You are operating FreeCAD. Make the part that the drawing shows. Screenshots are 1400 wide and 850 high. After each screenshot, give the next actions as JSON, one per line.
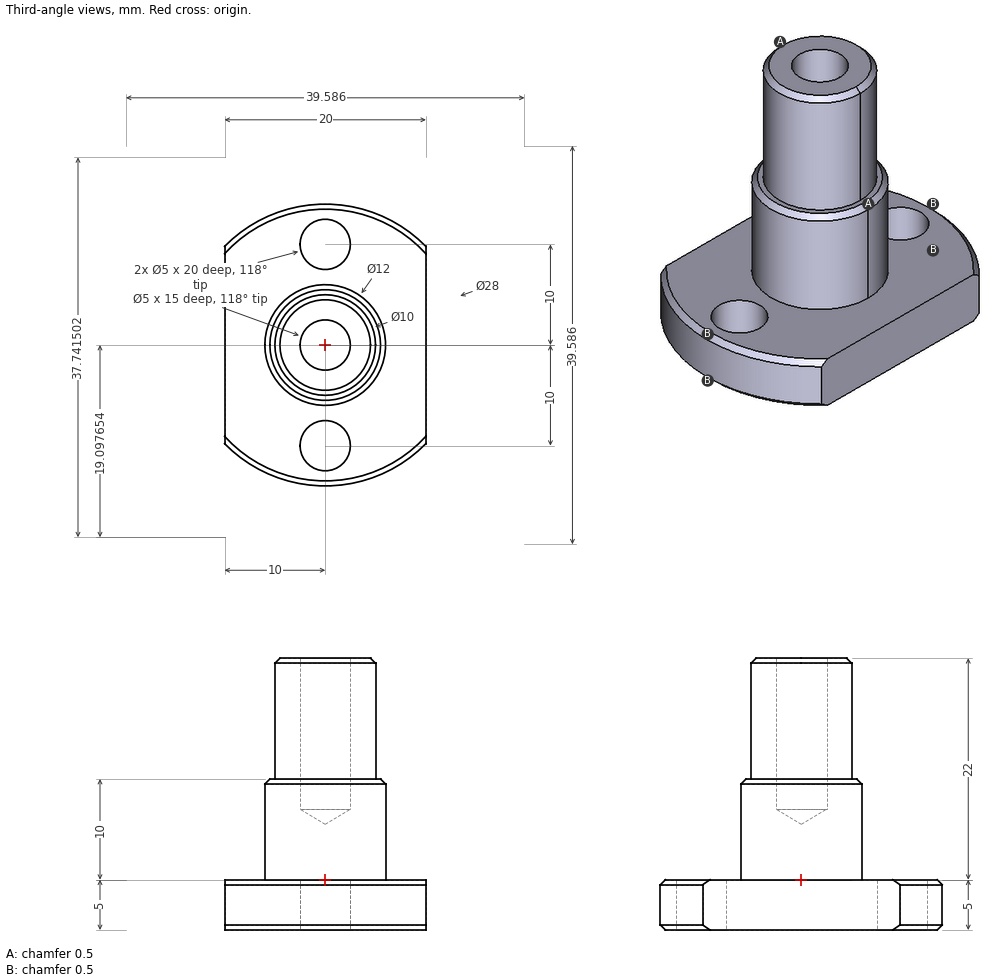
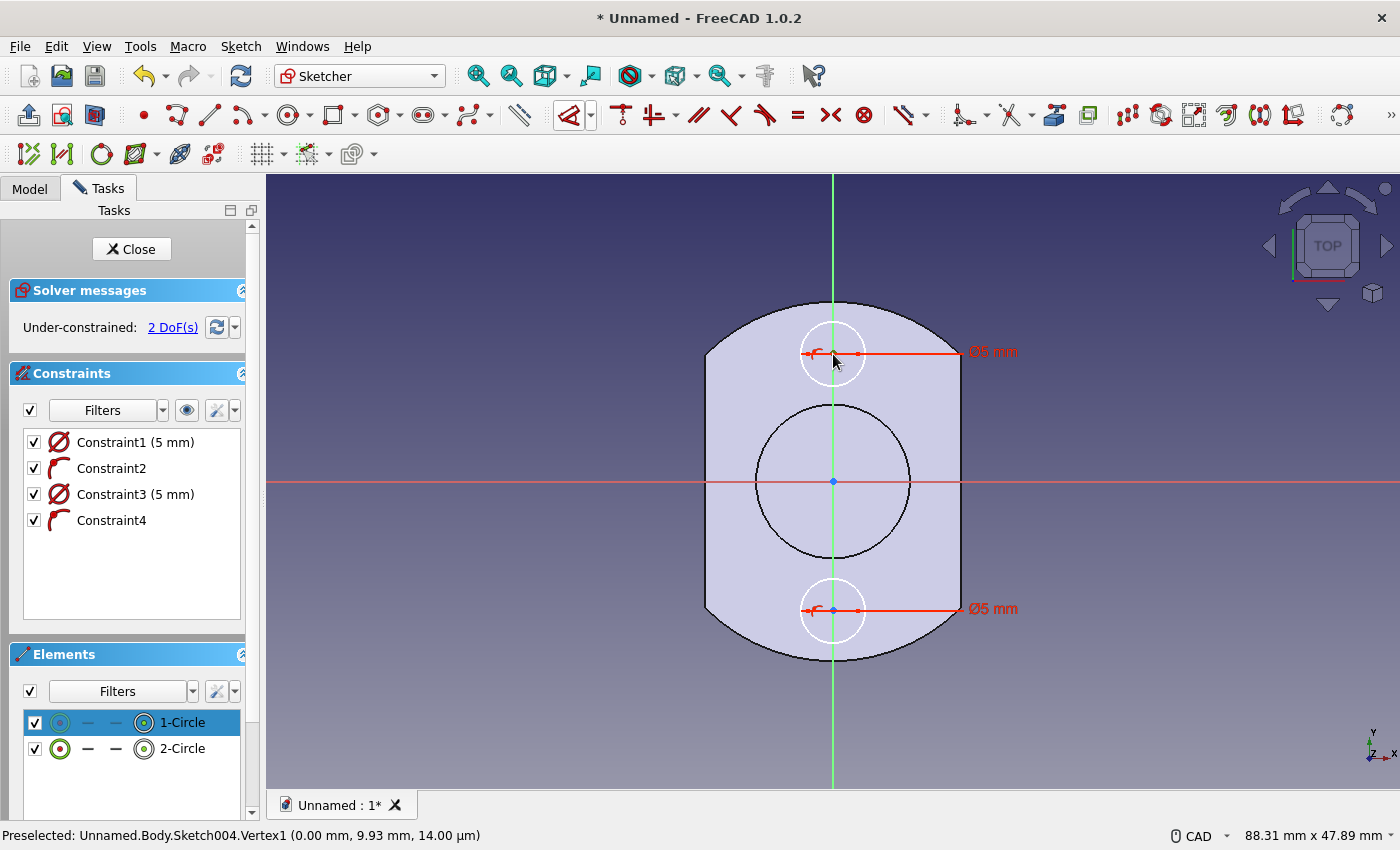
{"action": "key", "text": "i"}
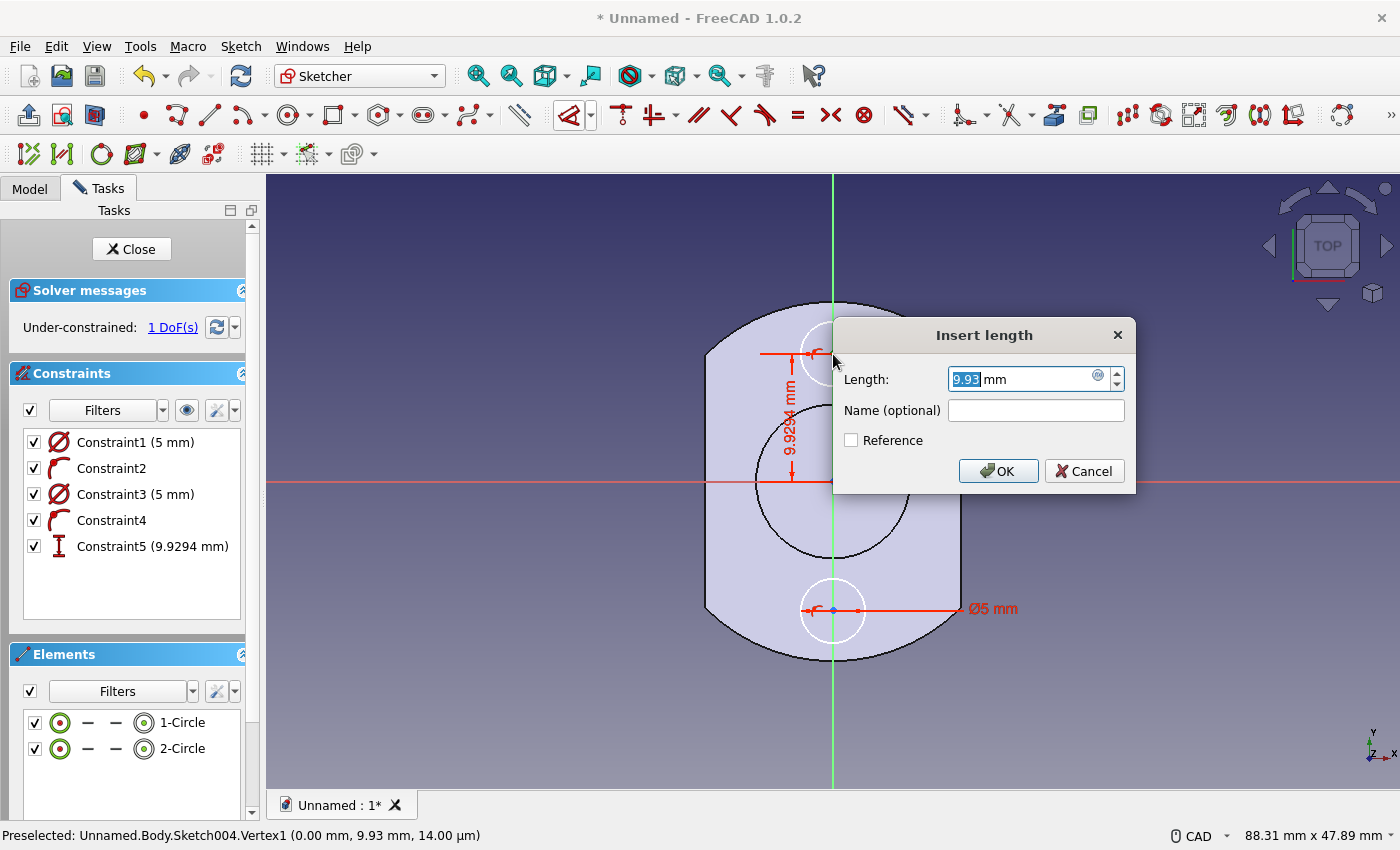
{"action": "type", "text": "10"}
{"action": "key", "text": "Return"}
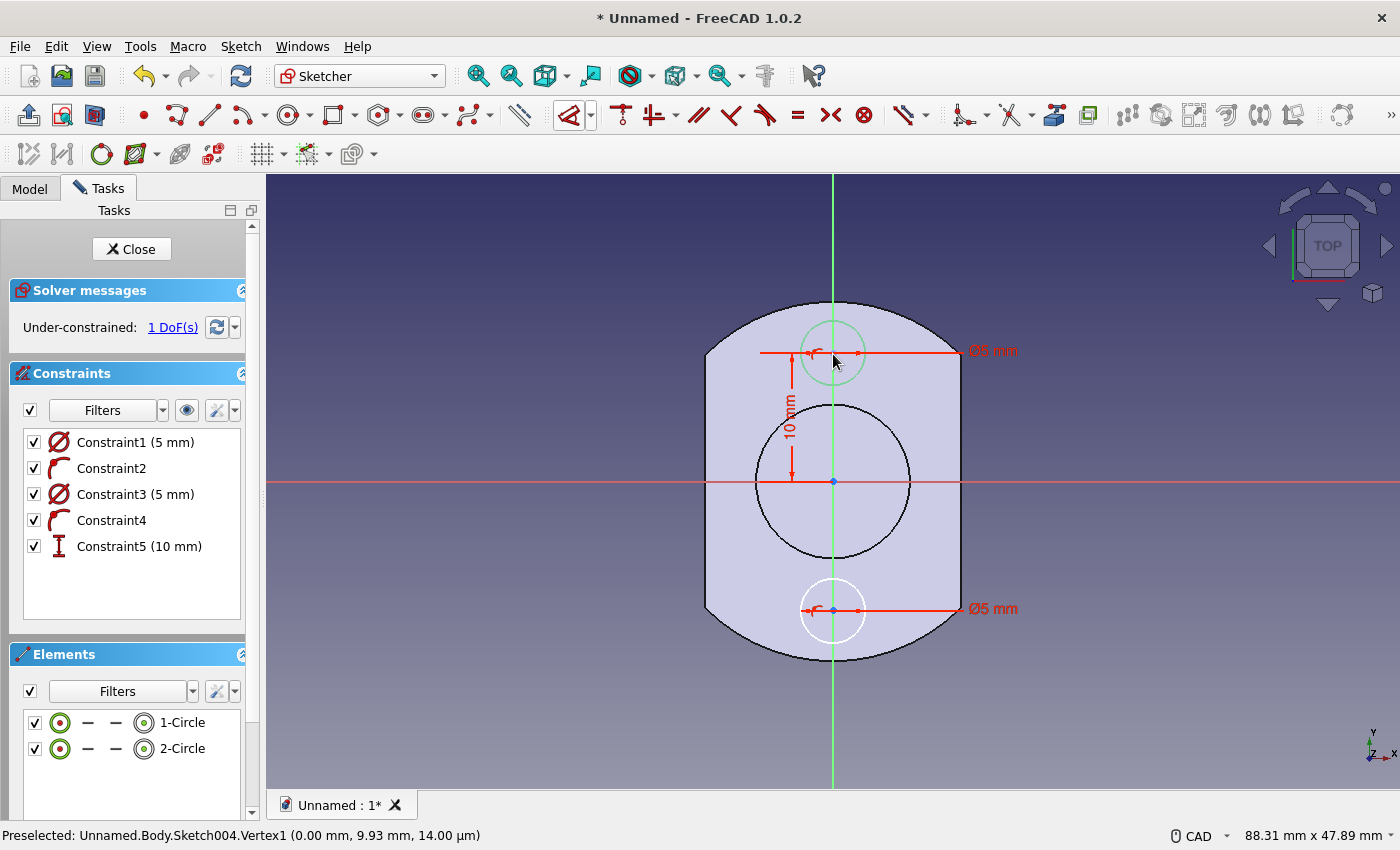
{"action": "left_click", "coordinate": [833, 611]}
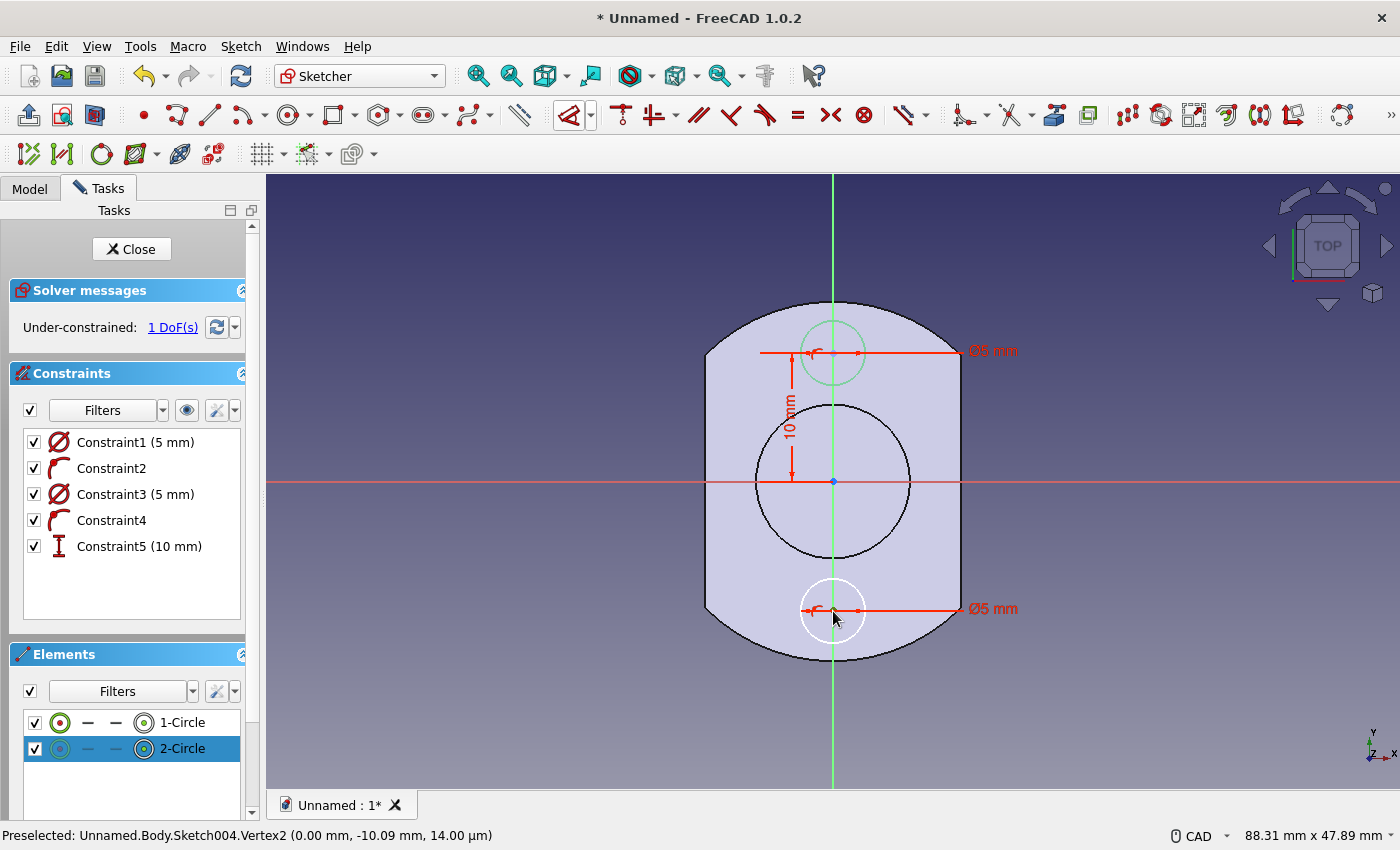
{"action": "key", "text": "i"}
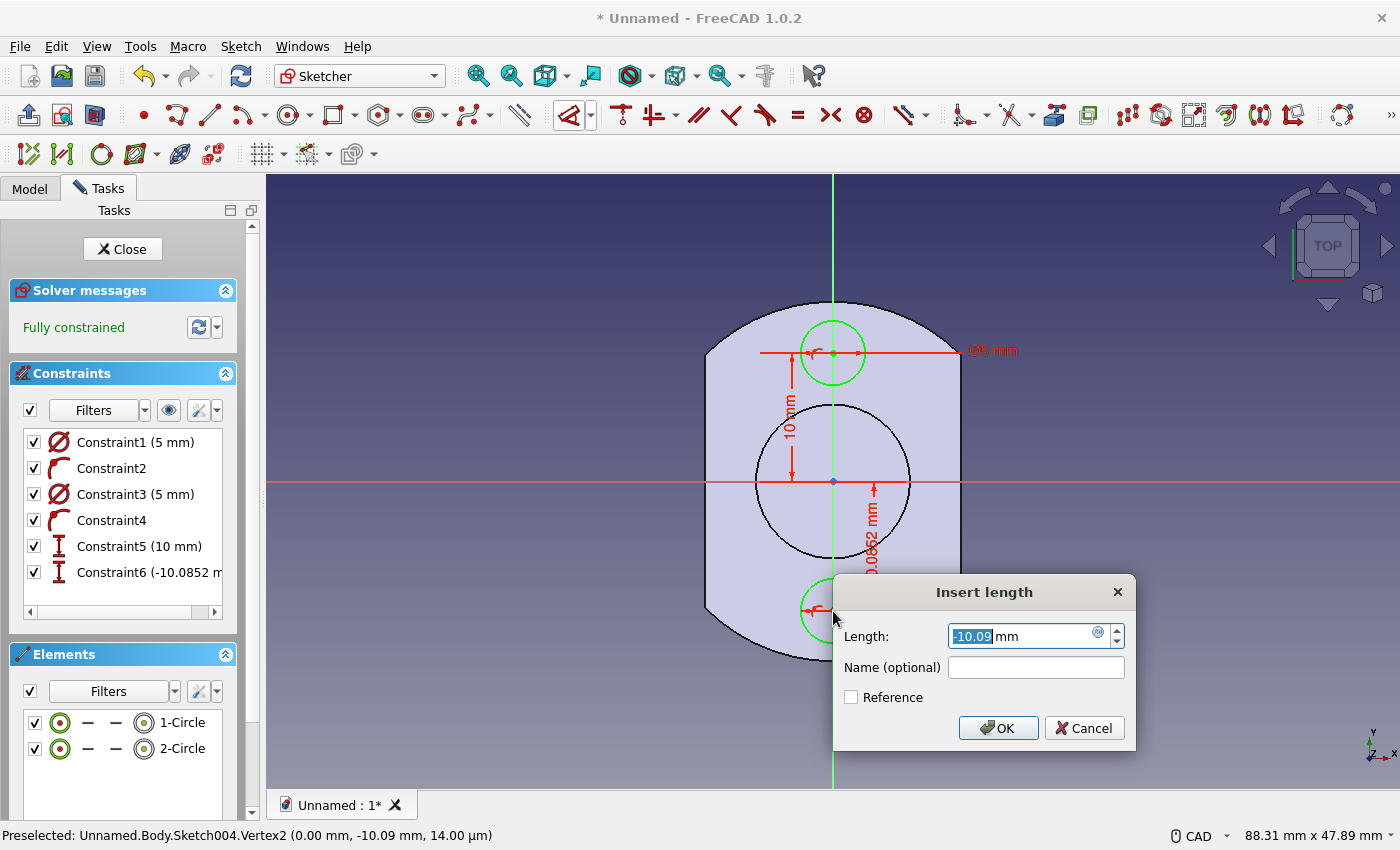
{"action": "type", "text": "-10"}
{"action": "key", "text": "Return"}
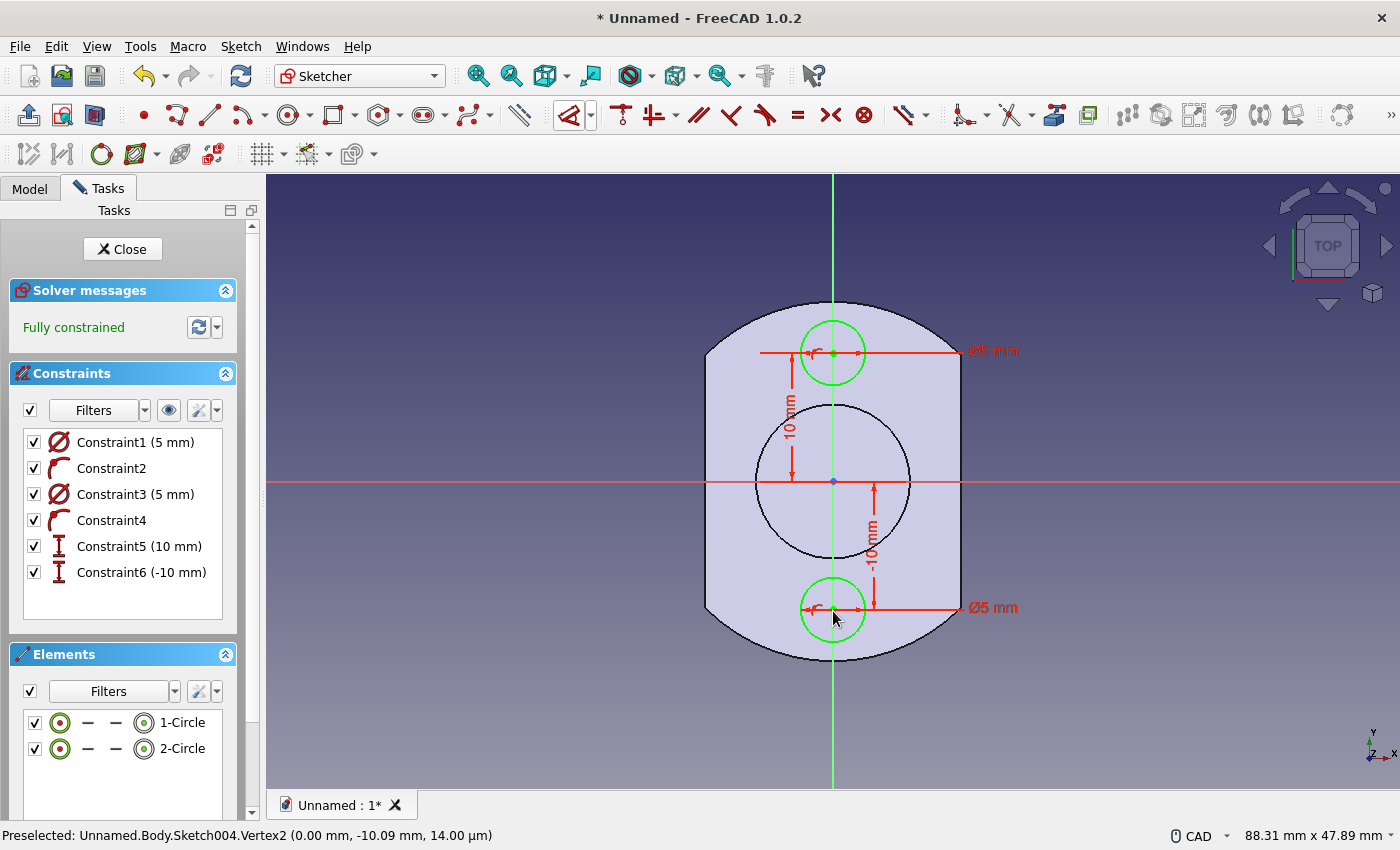
{"action": "left_click", "coordinate": [123, 249]}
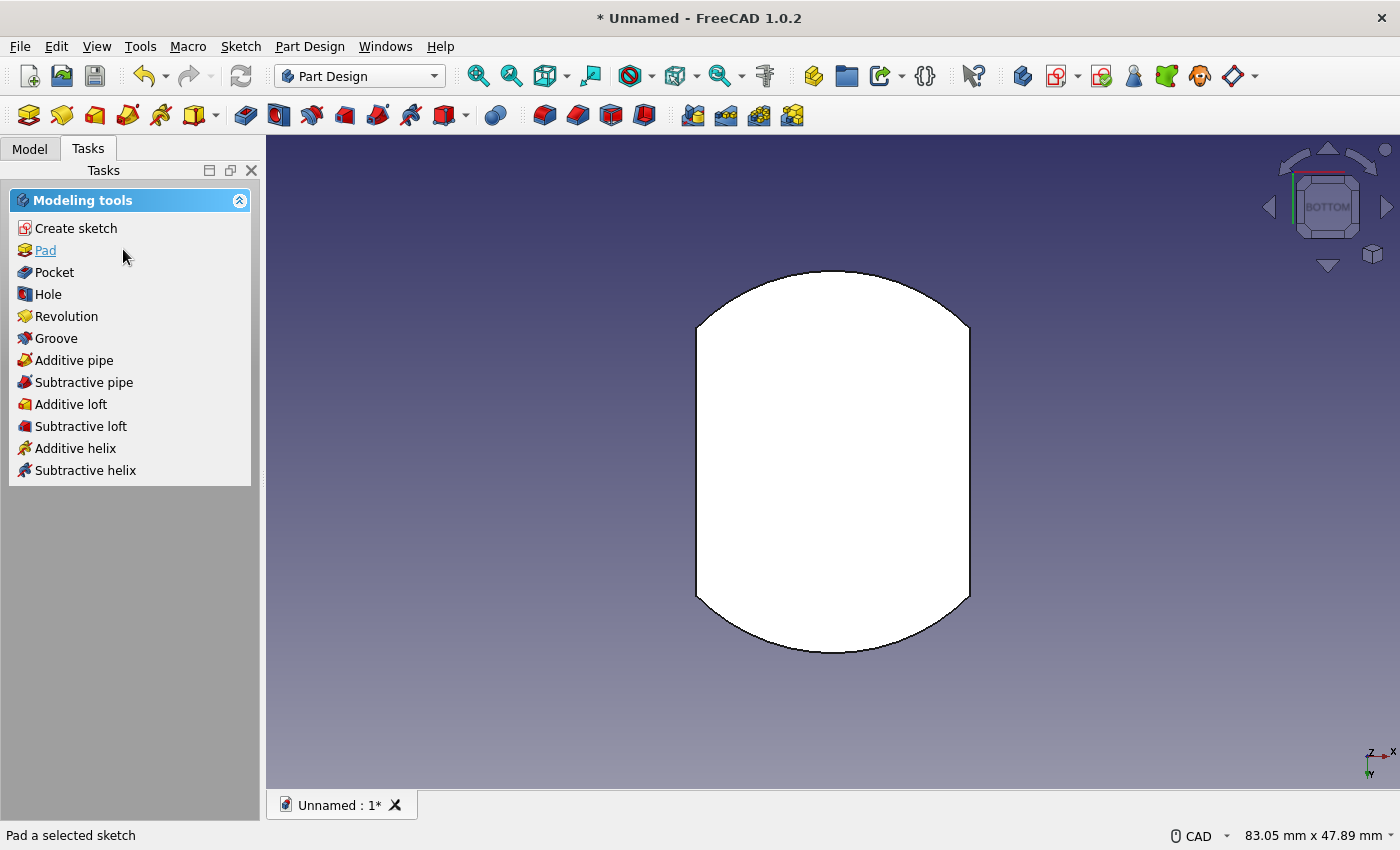
{"action": "left_click", "coordinate": [279, 116]}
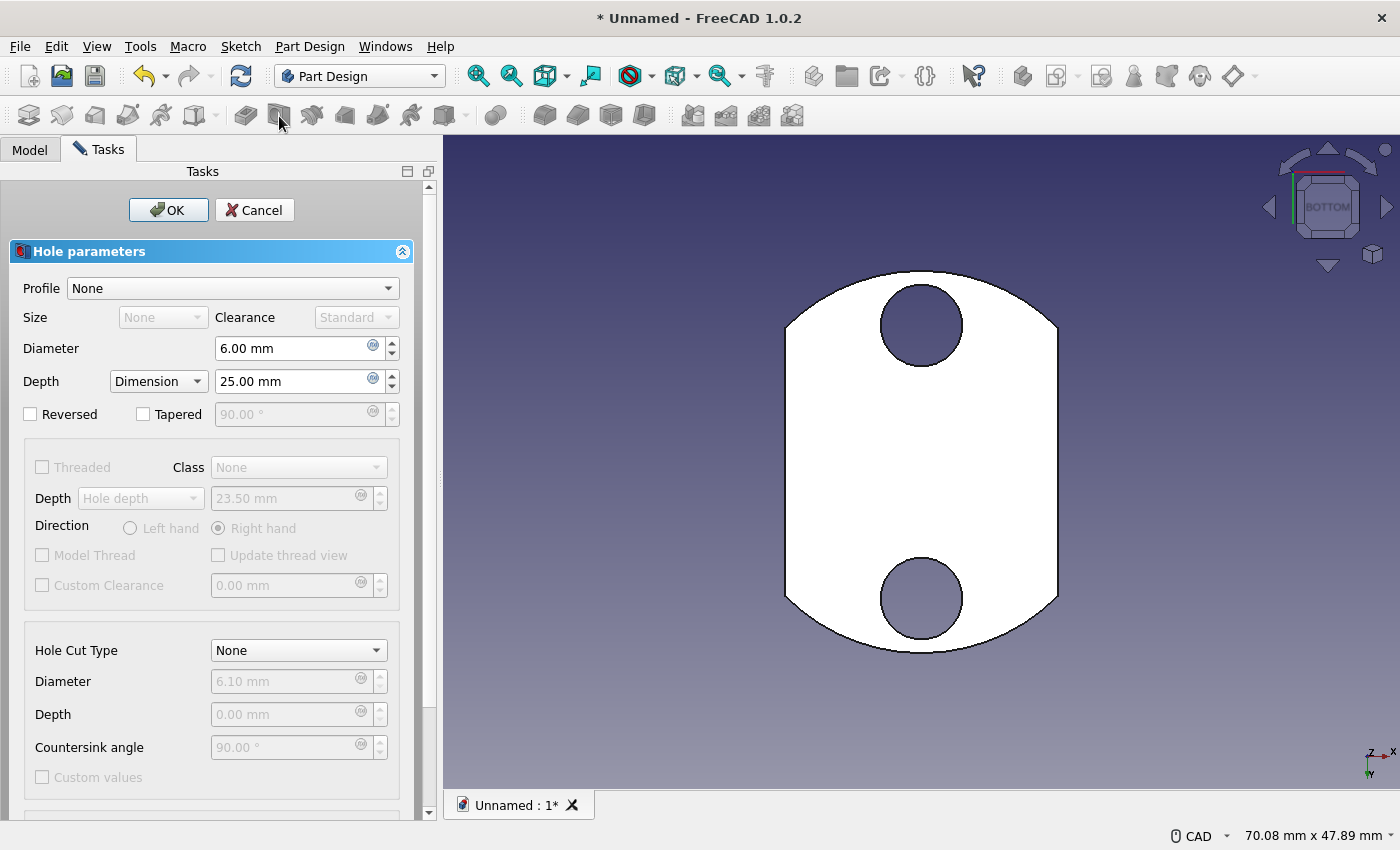
{"action": "triple_click", "coordinate": [300, 348]}